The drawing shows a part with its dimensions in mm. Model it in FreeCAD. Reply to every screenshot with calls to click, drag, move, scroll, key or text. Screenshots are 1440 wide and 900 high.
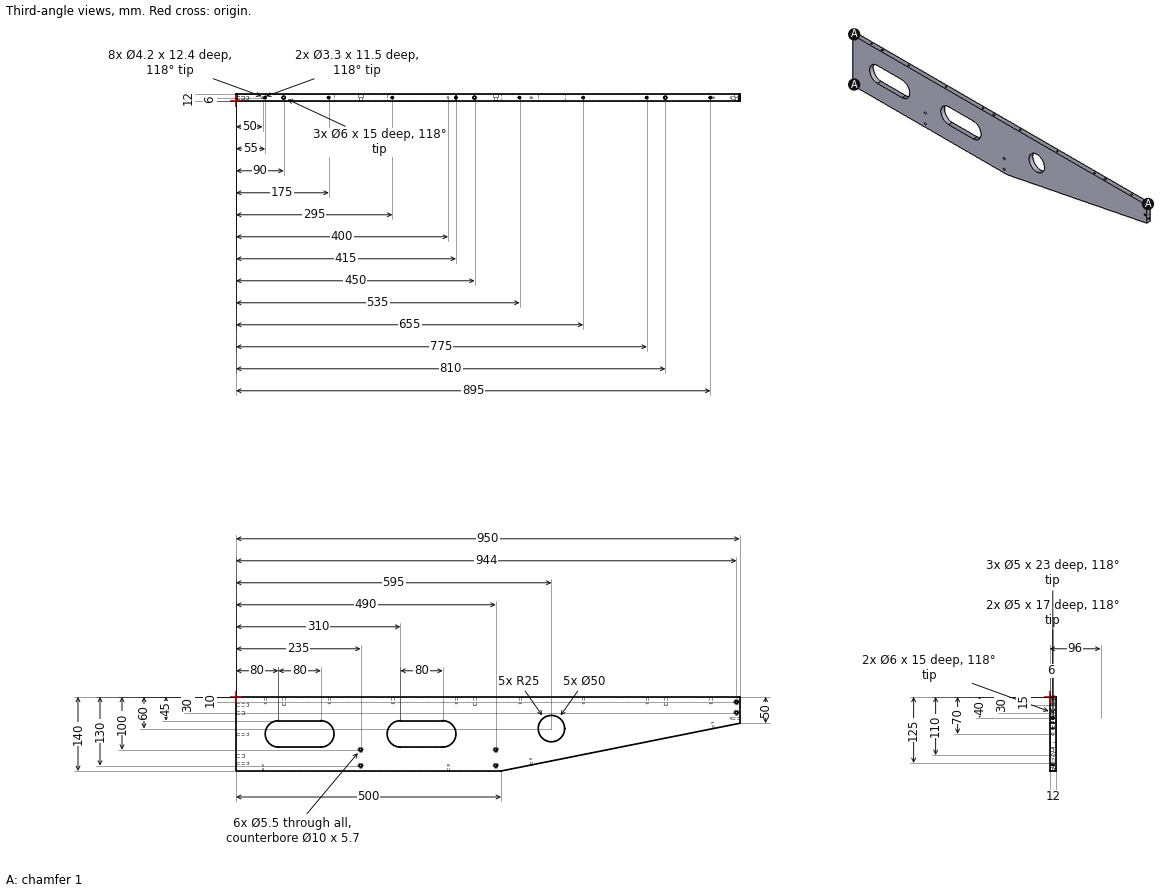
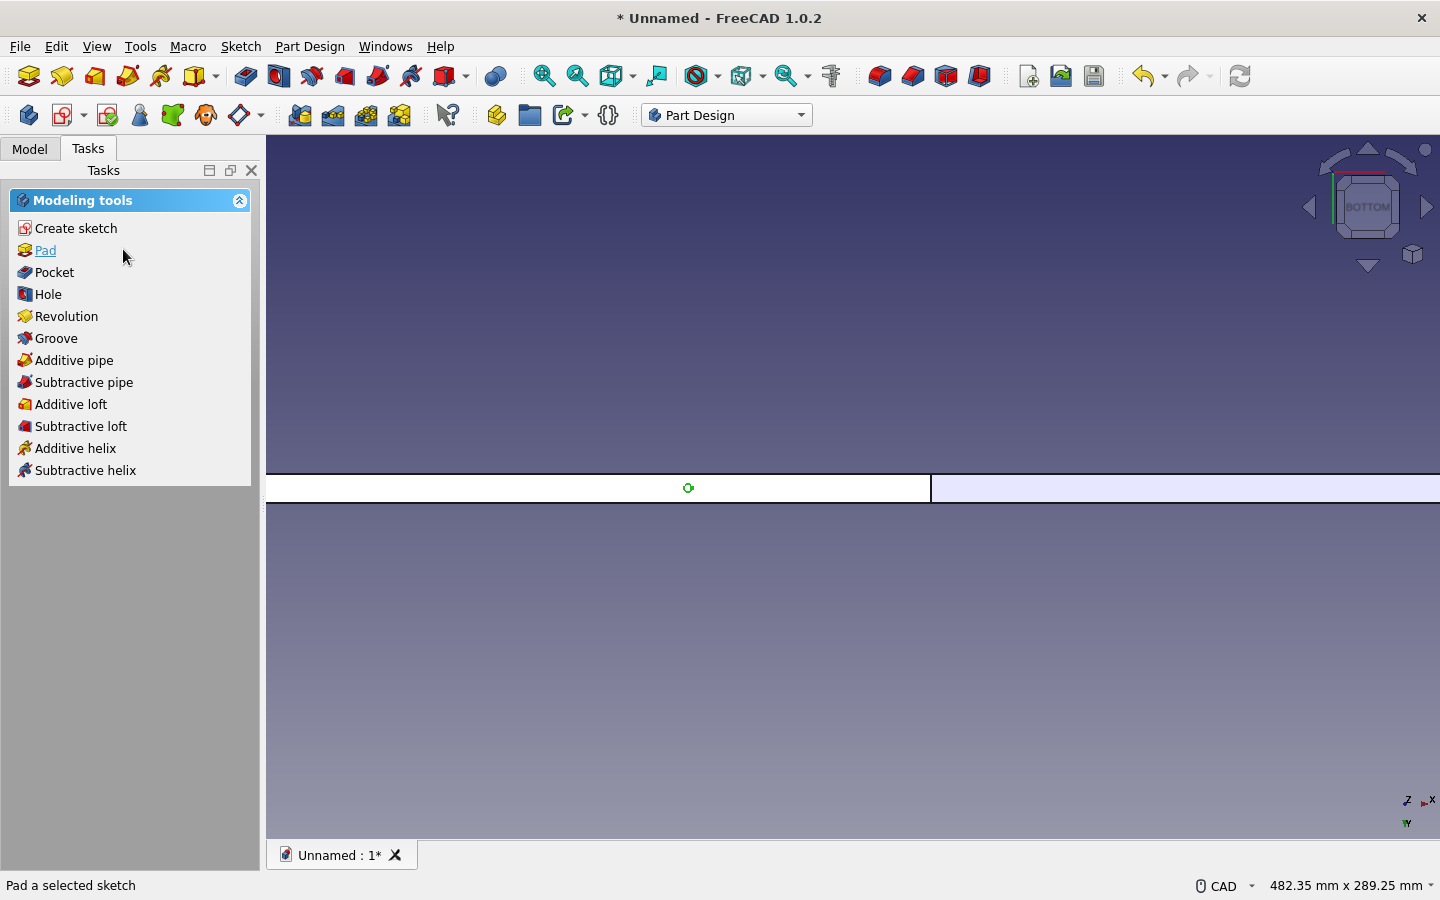
click(279, 76)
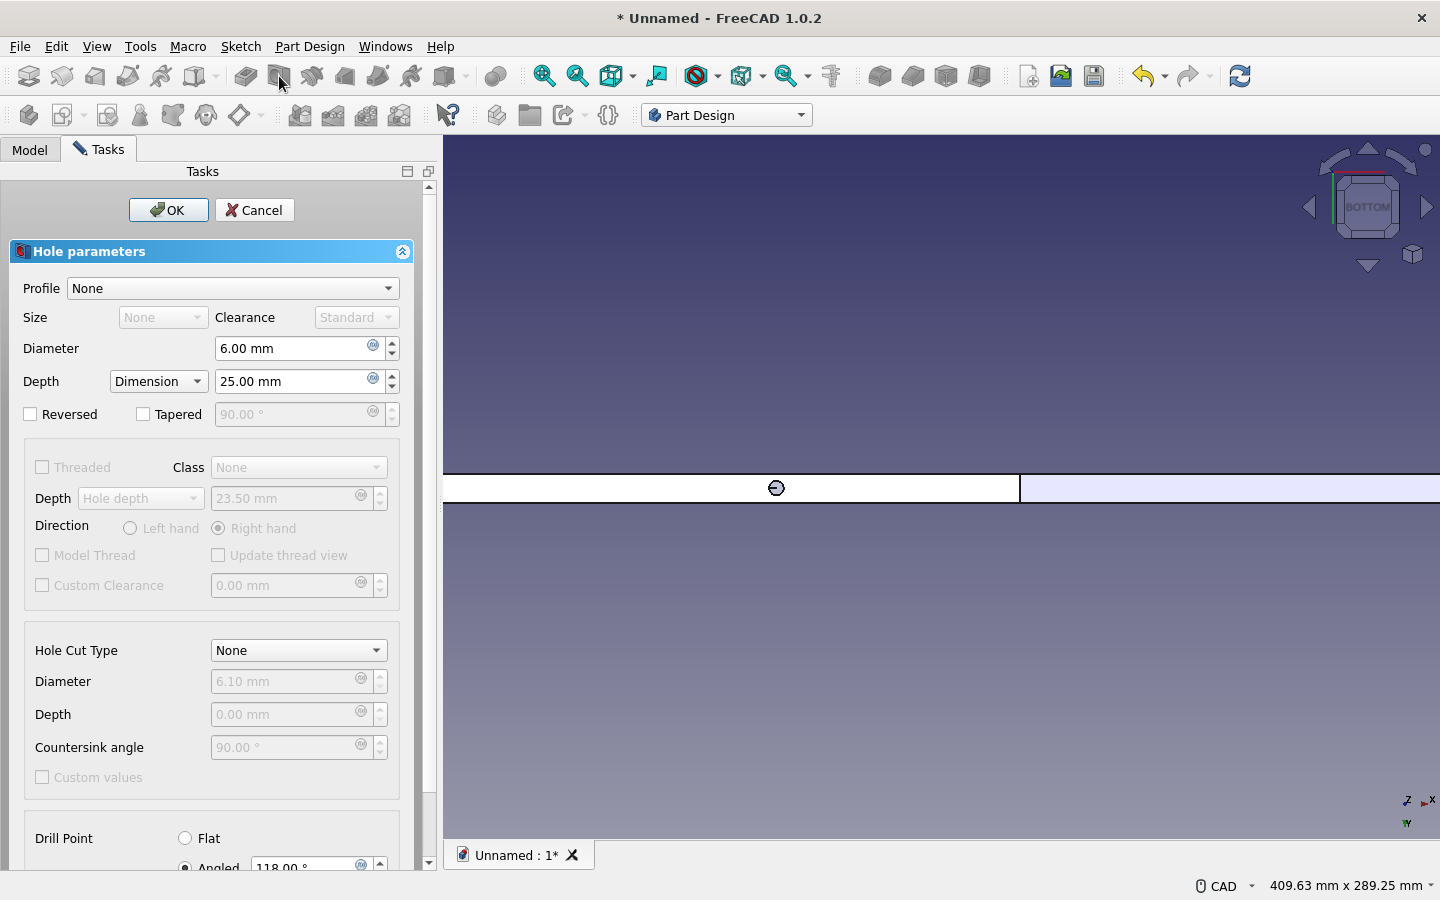
triple_click(300, 348)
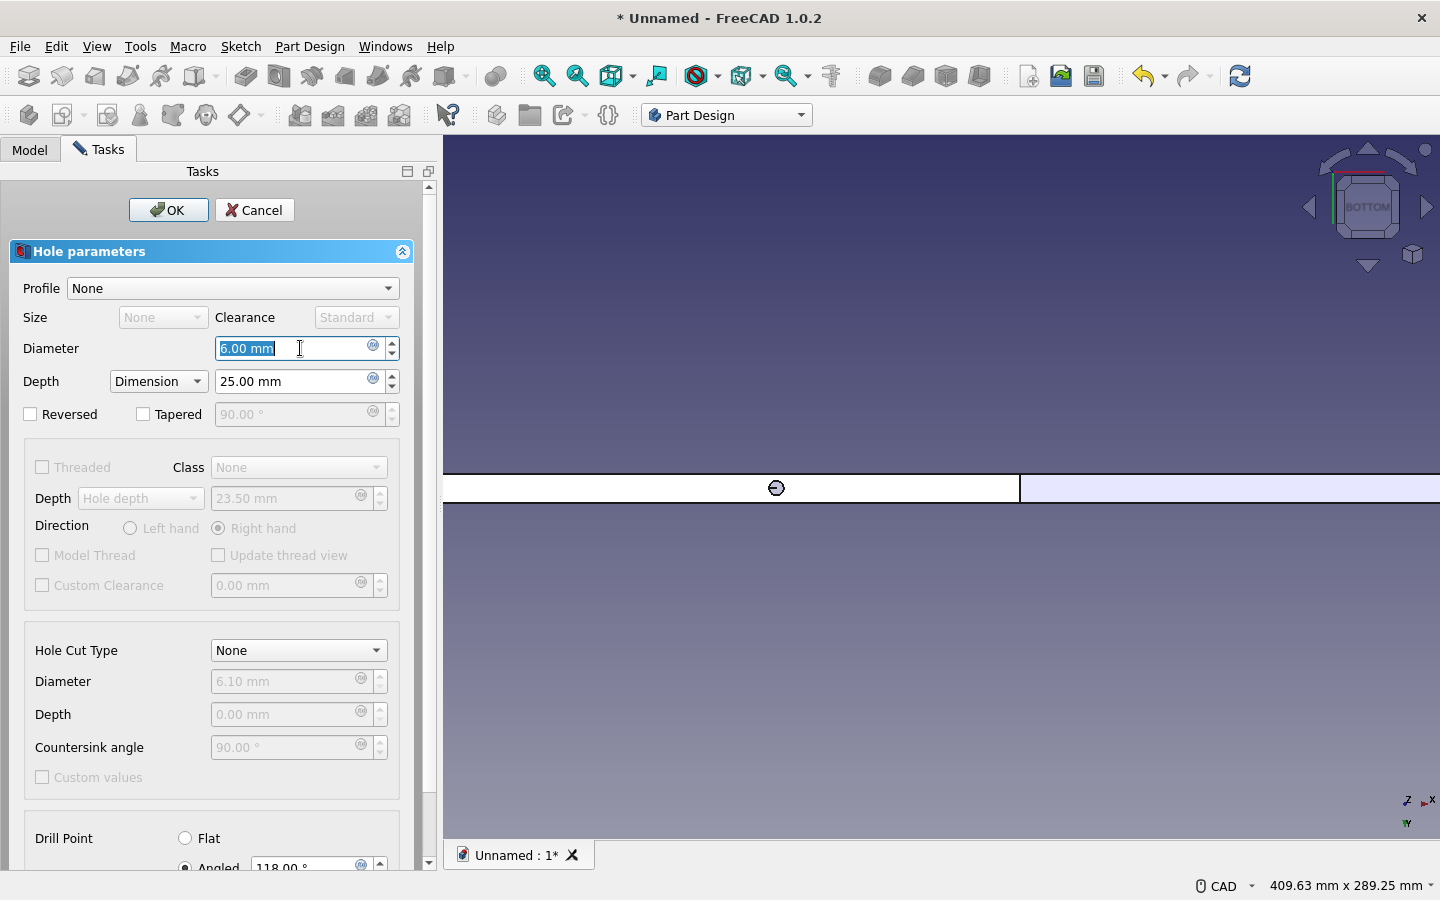
text(3.3)
key(Tab)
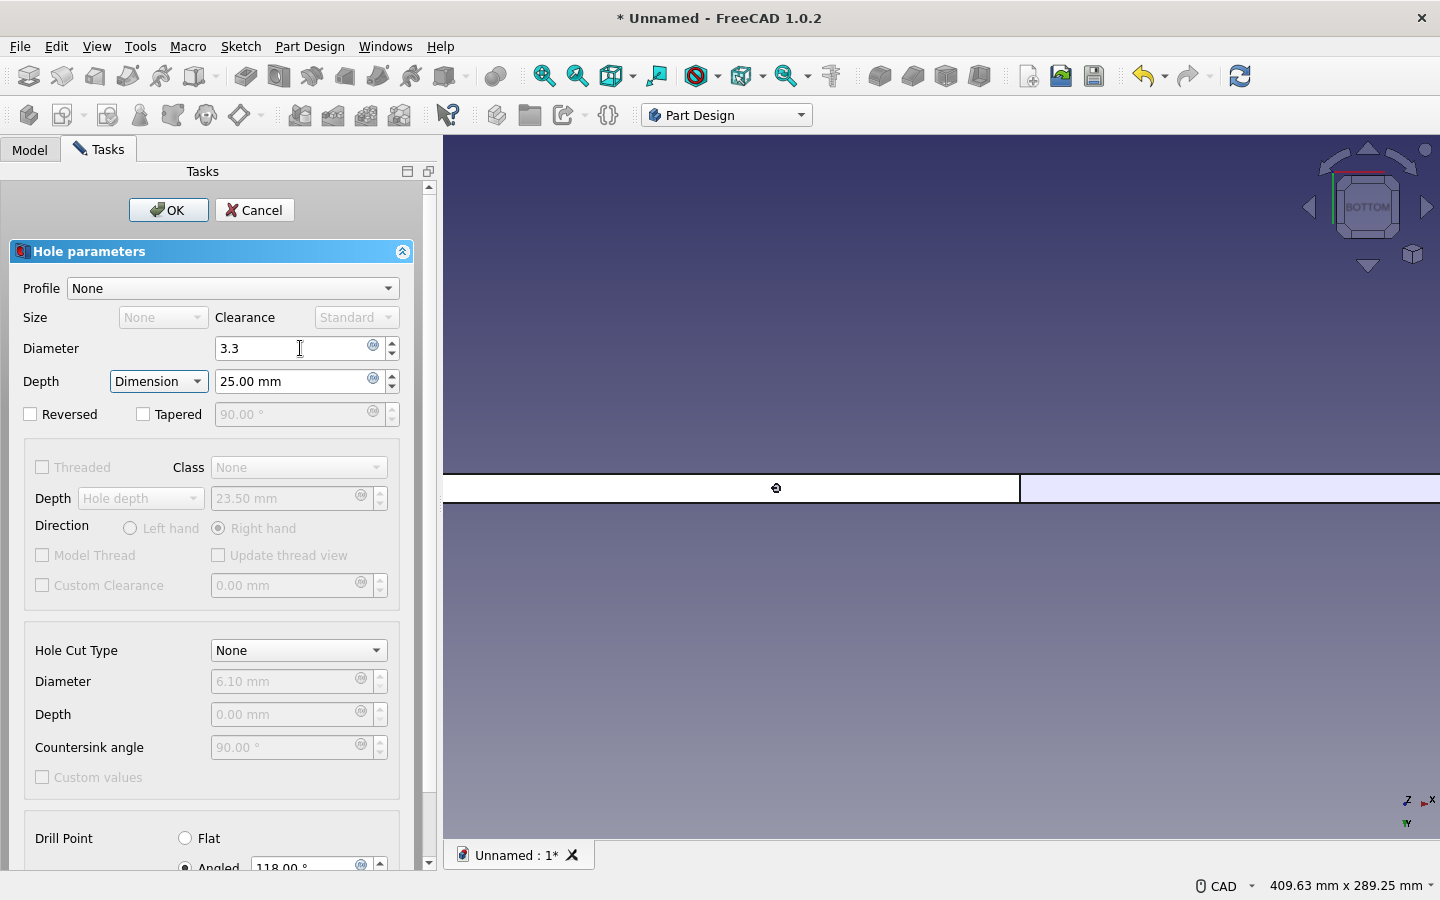
triple_click(300, 382)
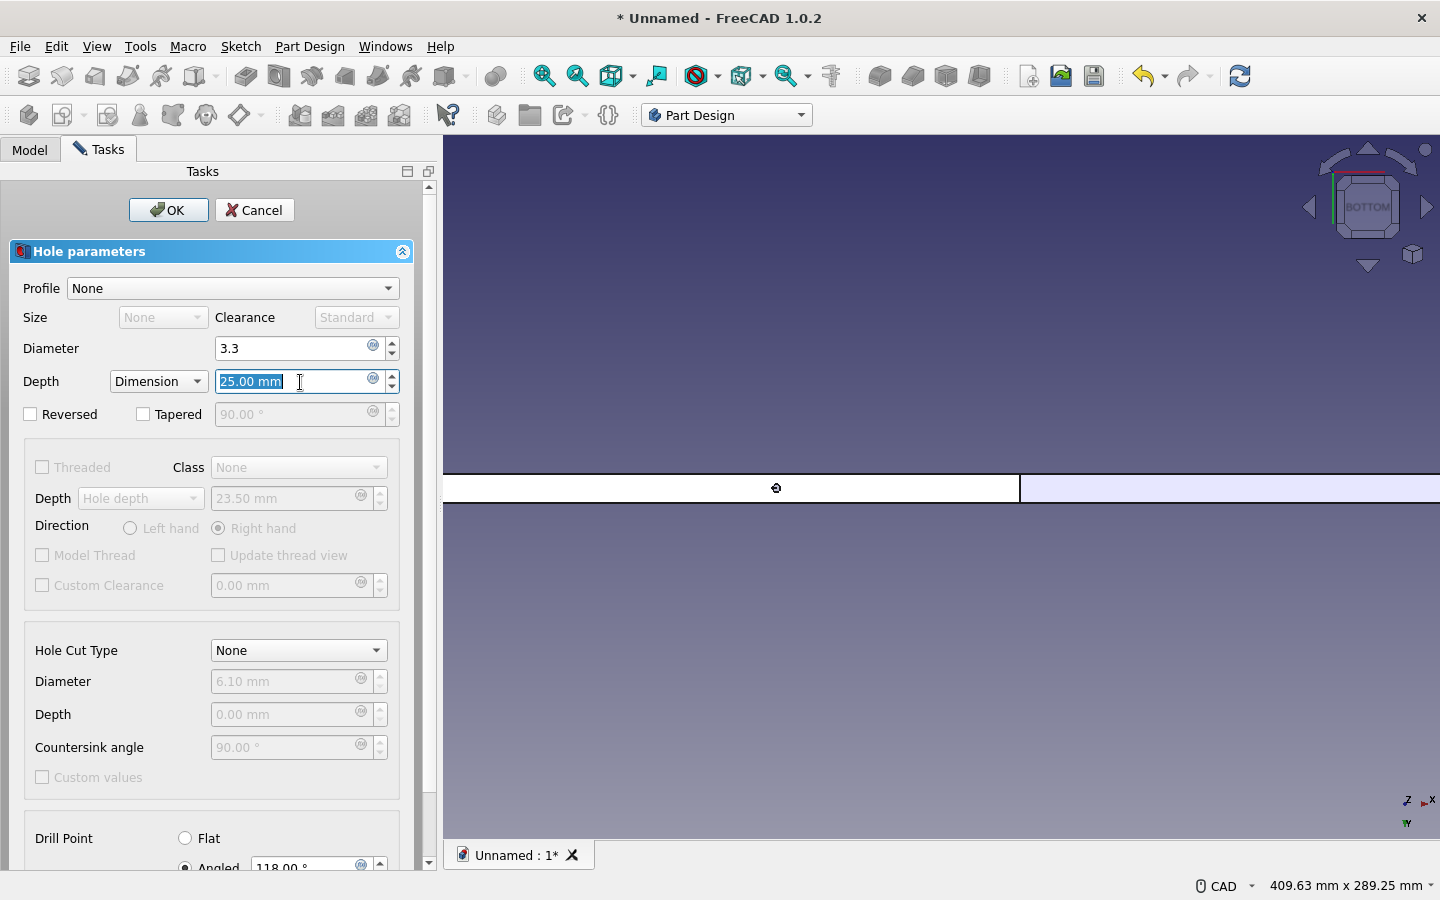
text(11.5)
key(Tab)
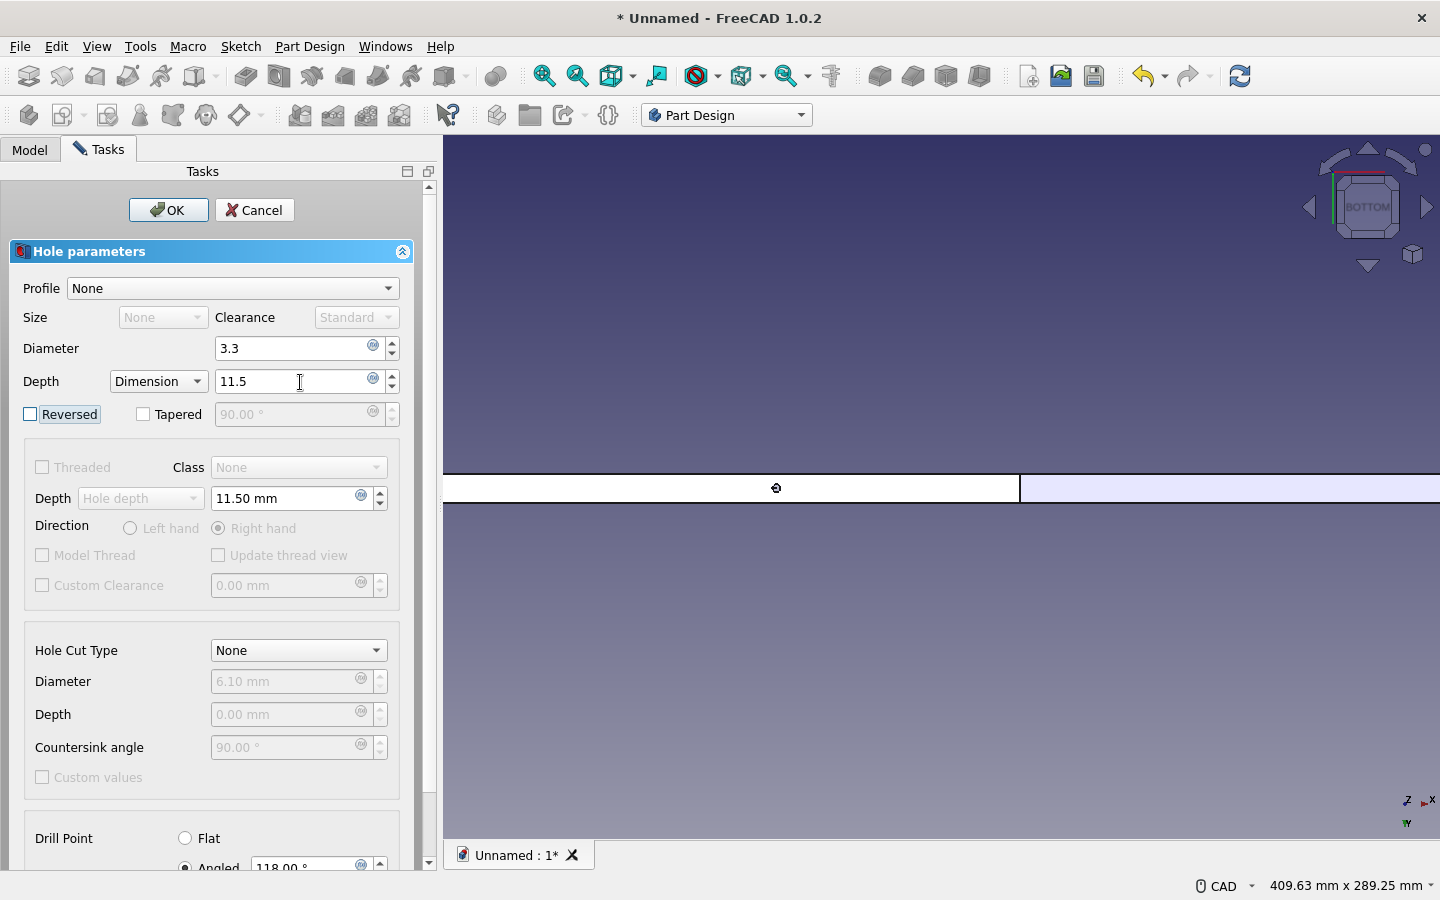
click(169, 210)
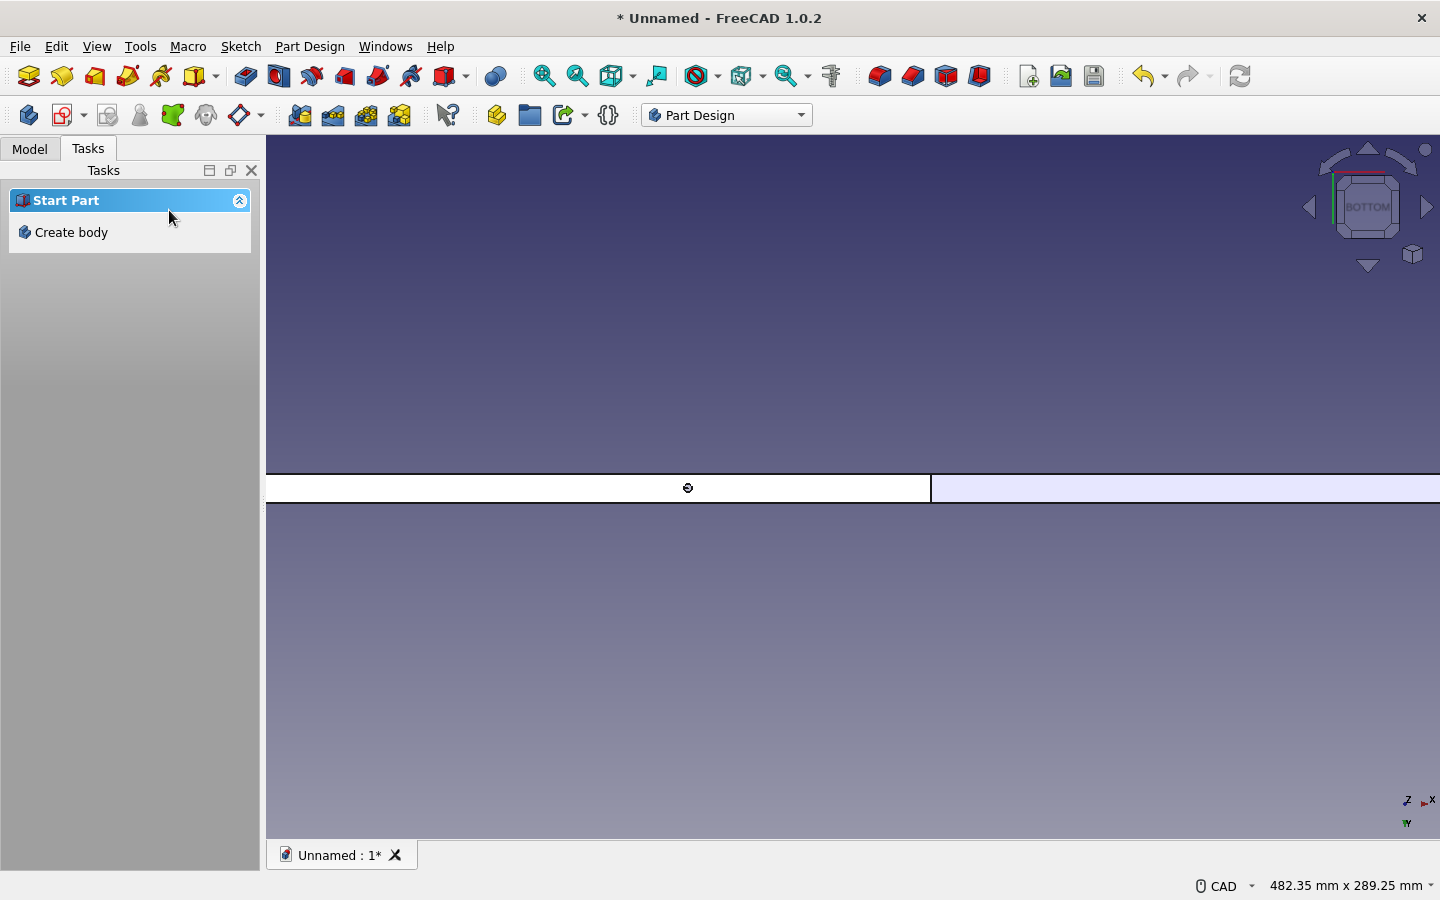
click(545, 76)